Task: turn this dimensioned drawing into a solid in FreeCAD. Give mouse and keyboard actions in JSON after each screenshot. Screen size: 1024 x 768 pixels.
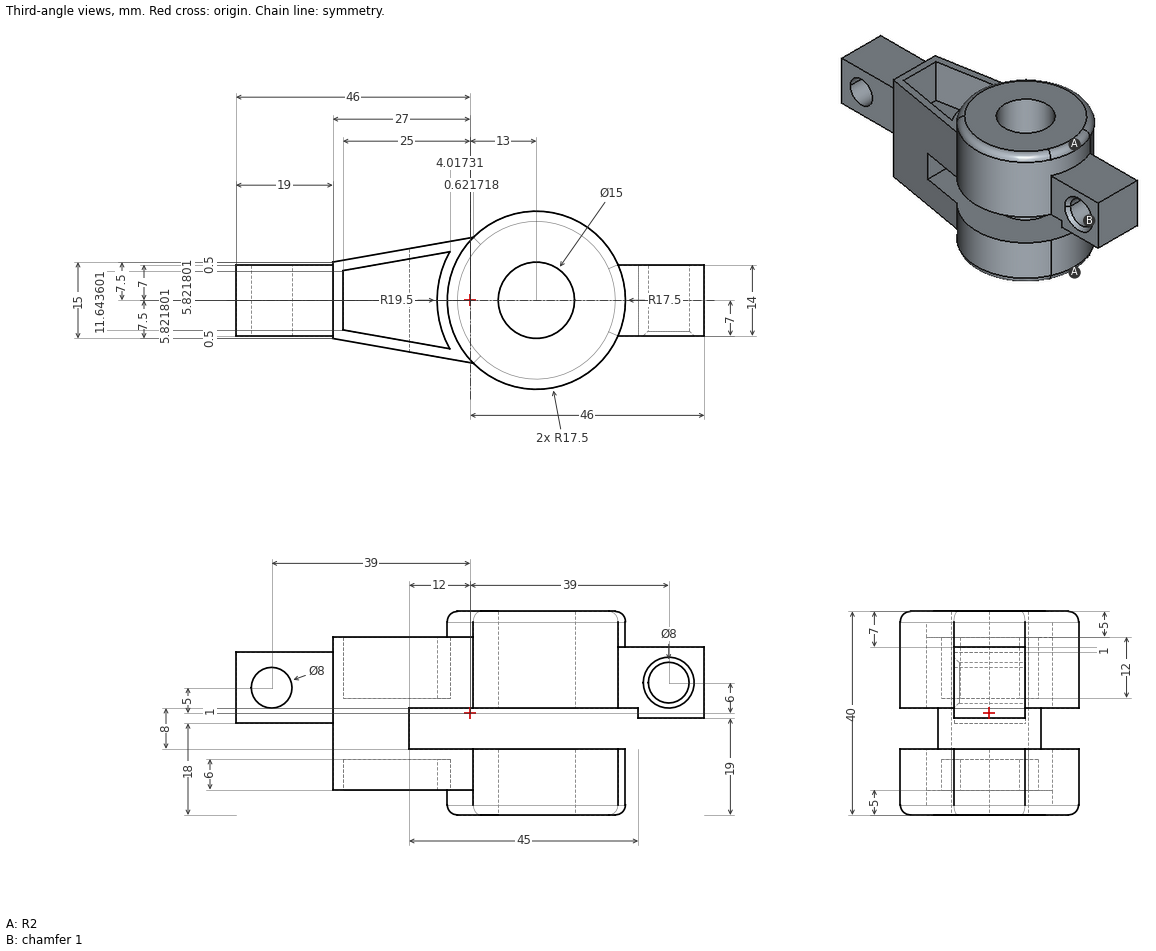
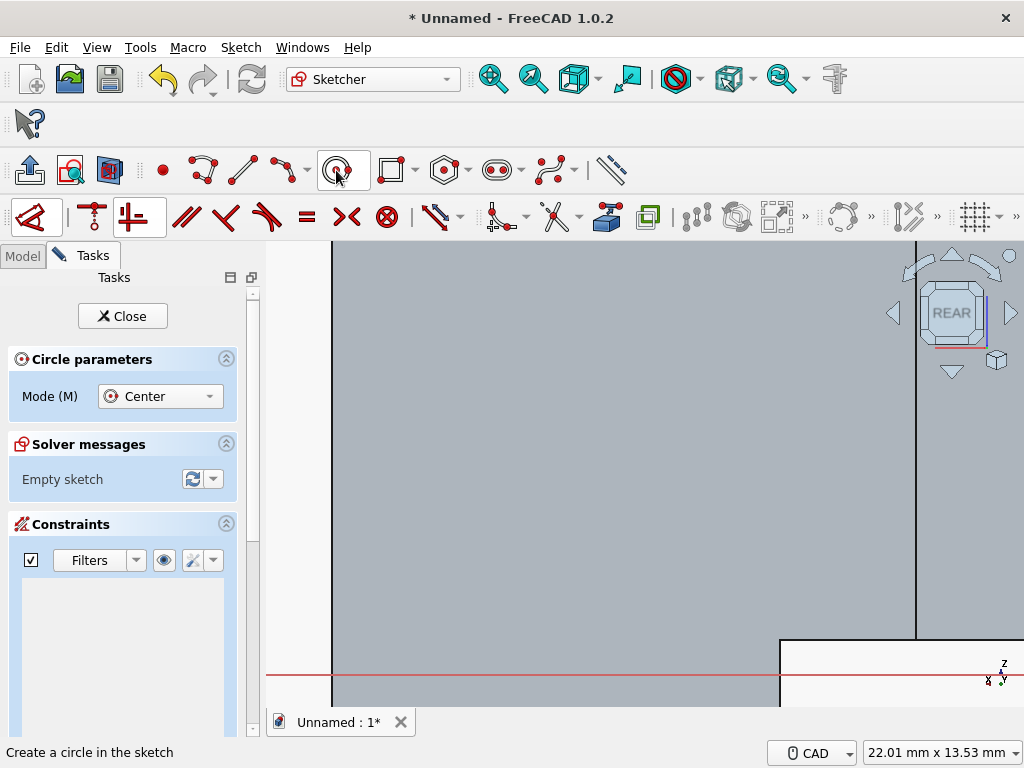
{"action": "left_click", "coordinate": [573, 468]}
{"action": "left_click", "coordinate": [670, 371]}
{"action": "key", "text": "Escape"}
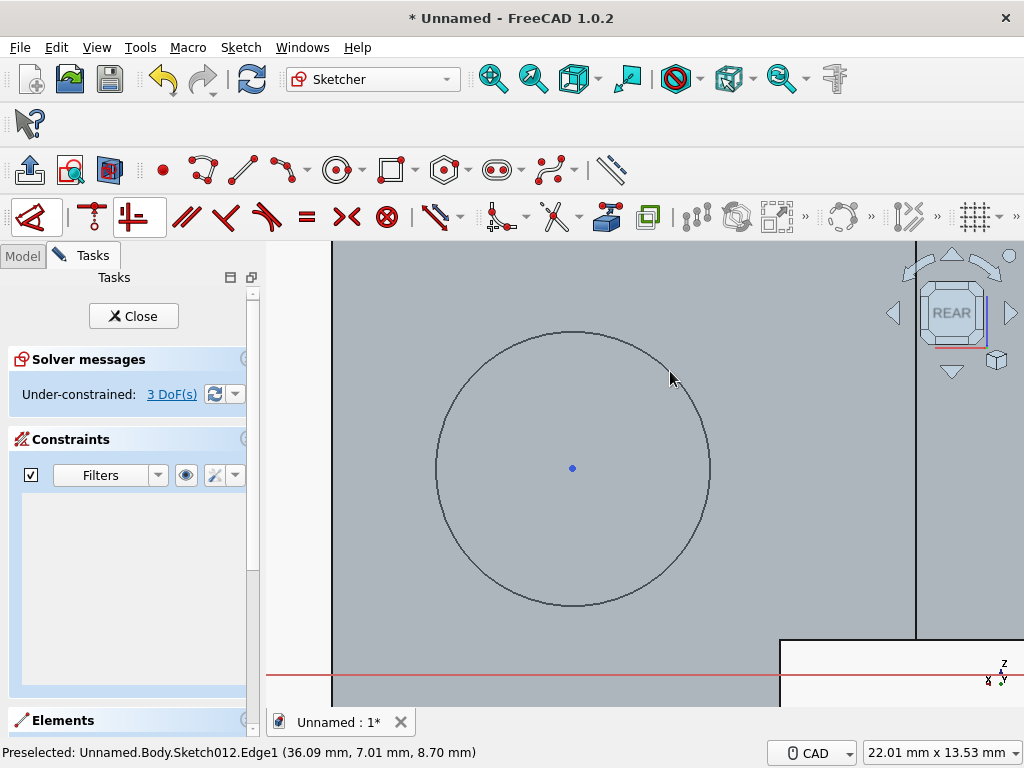
{"action": "left_click", "coordinate": [670, 372]}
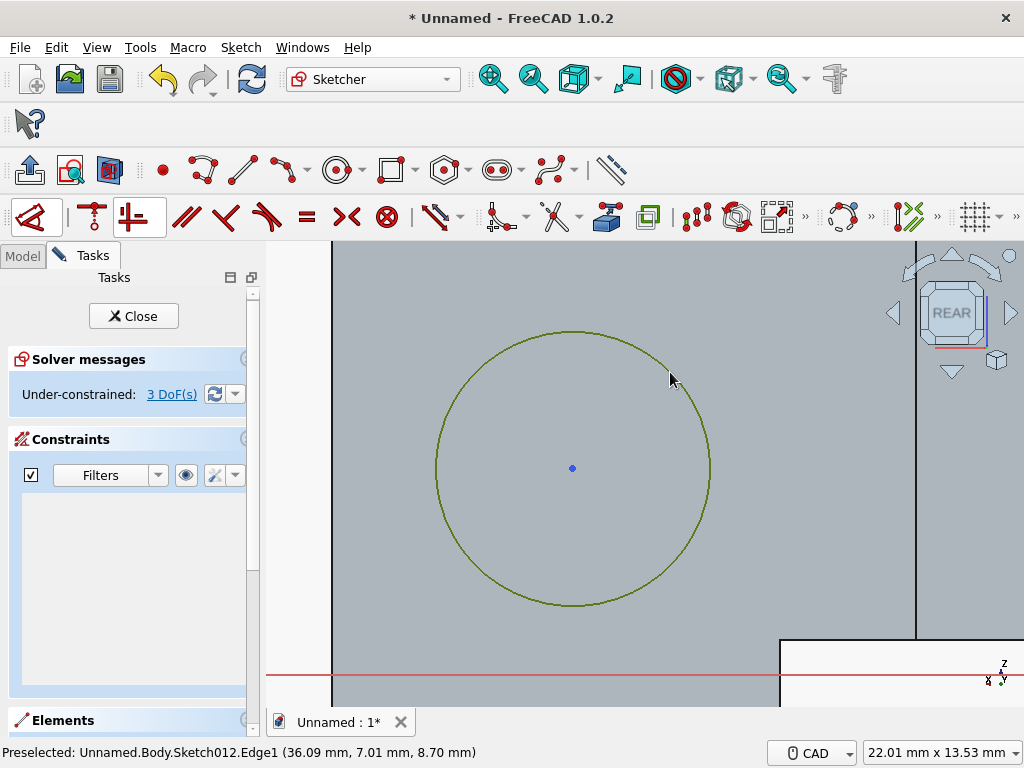
{"action": "key", "text": "k o"}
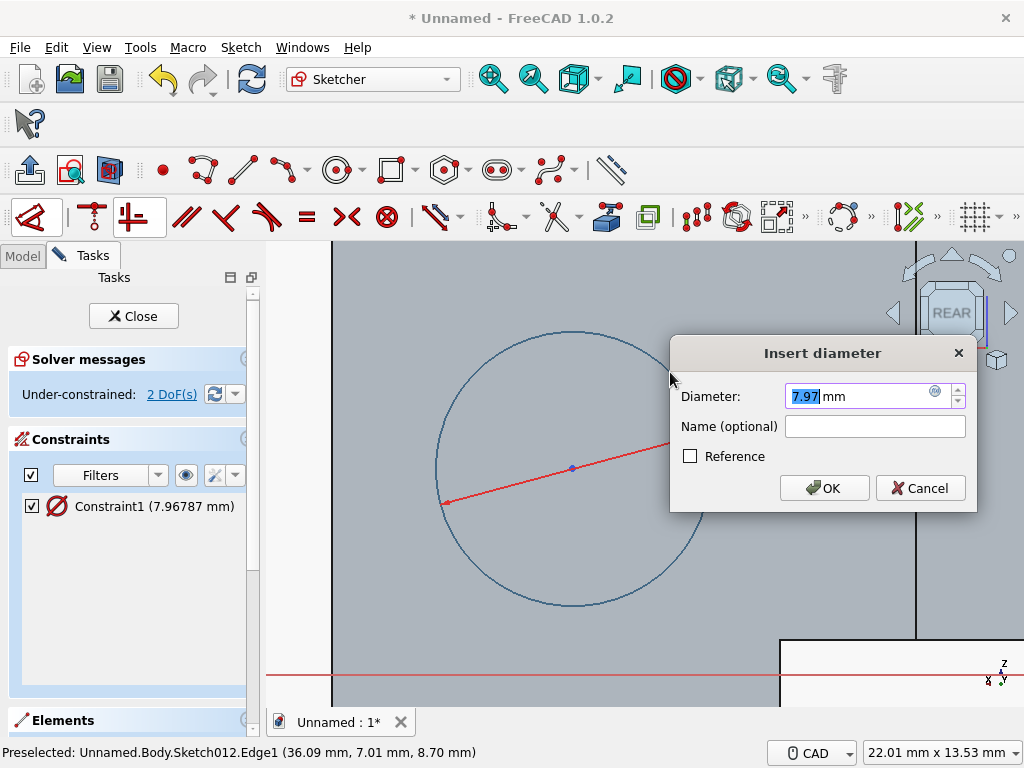
{"action": "type", "text": "8"}
{"action": "key", "text": "Return"}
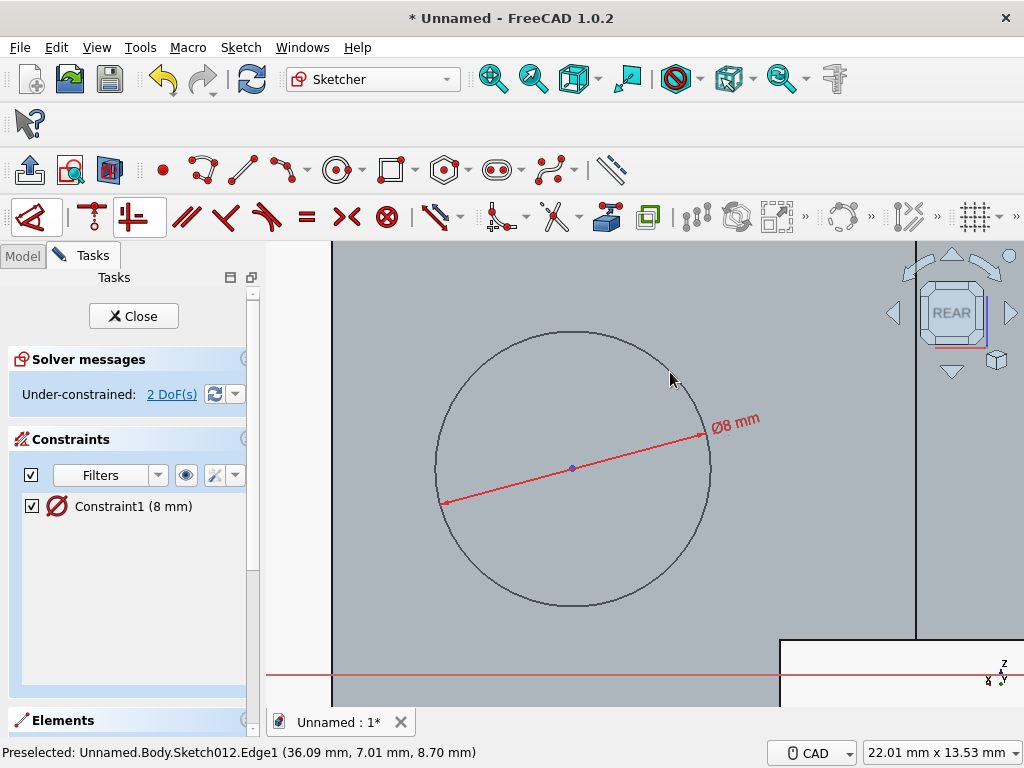
{"action": "left_click", "coordinate": [573, 469]}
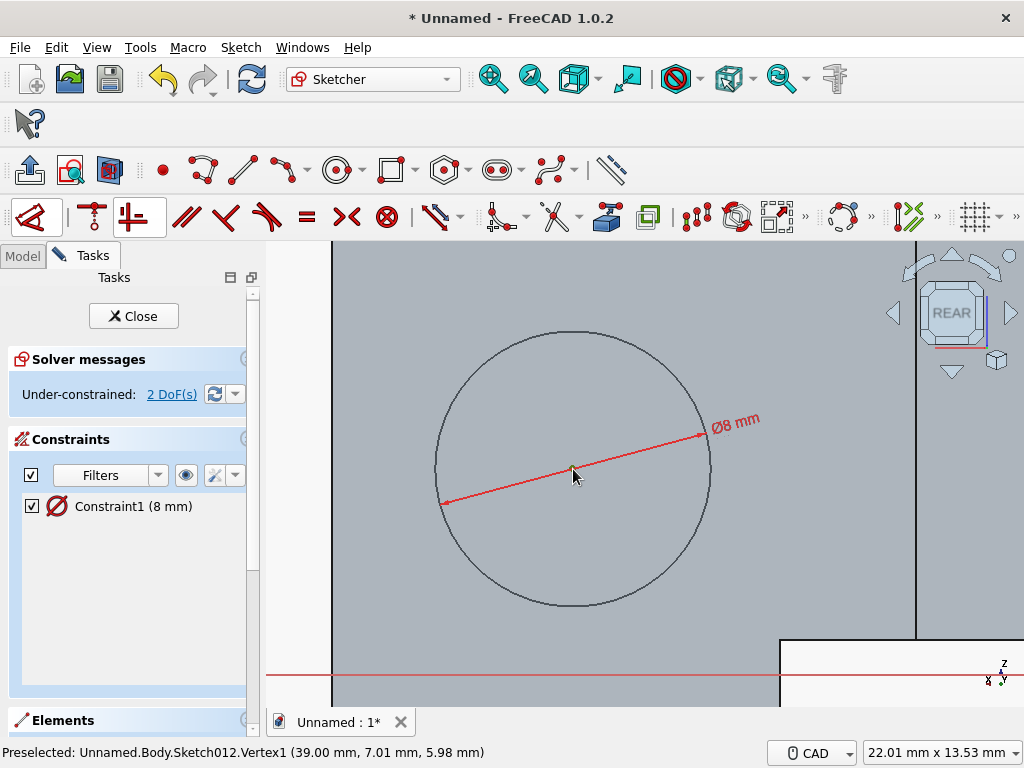
{"action": "key", "text": "i"}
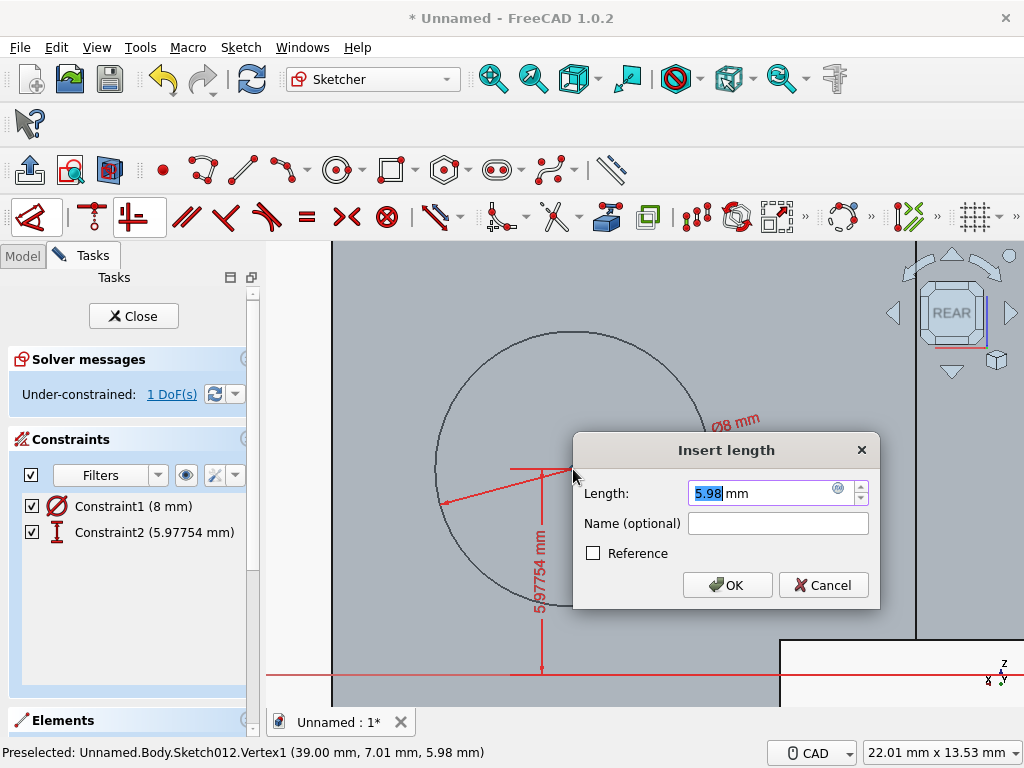
{"action": "type", "text": "6"}
{"action": "key", "text": "Return"}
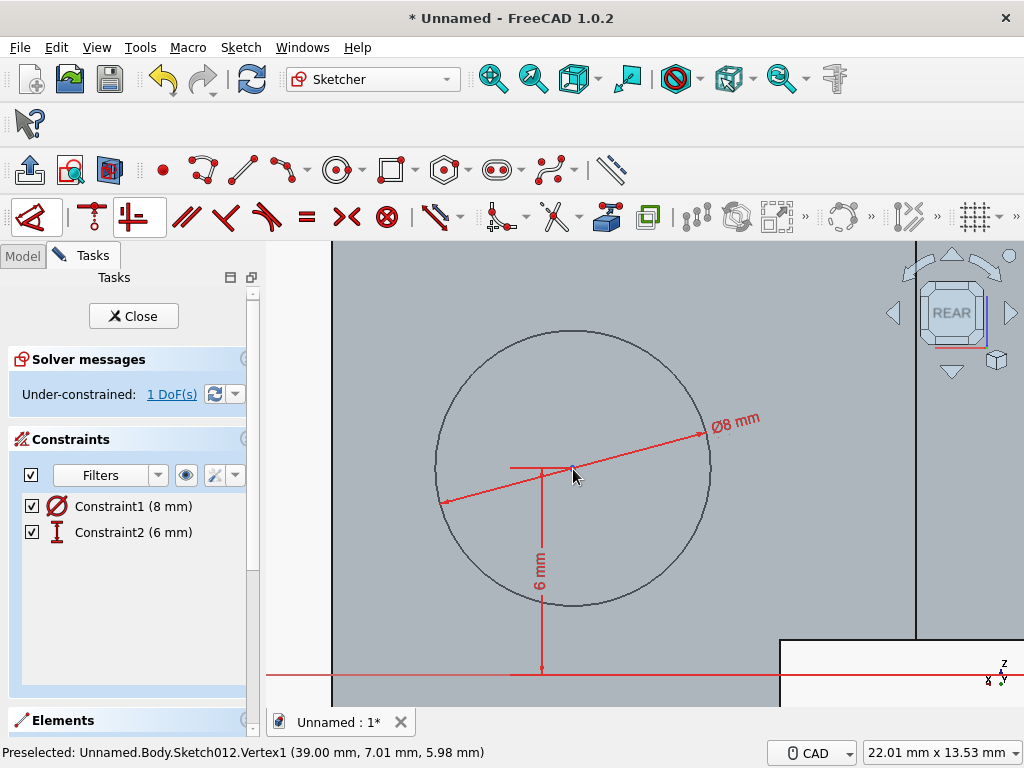
{"action": "left_click", "coordinate": [573, 468]}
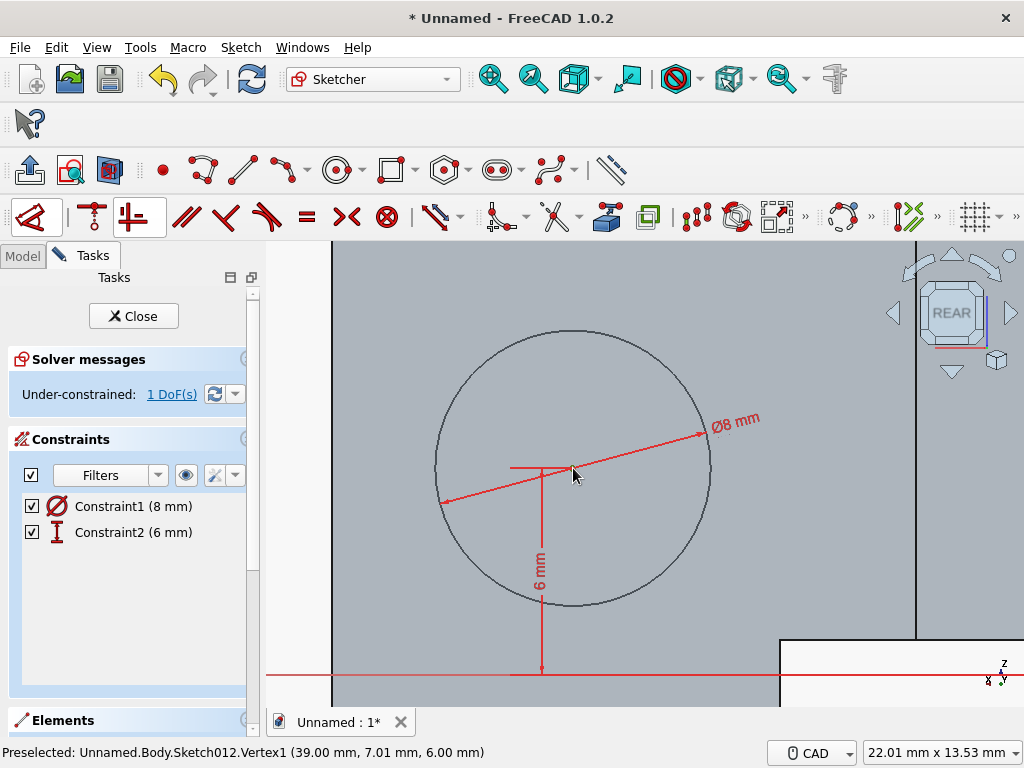
{"action": "key", "text": "l"}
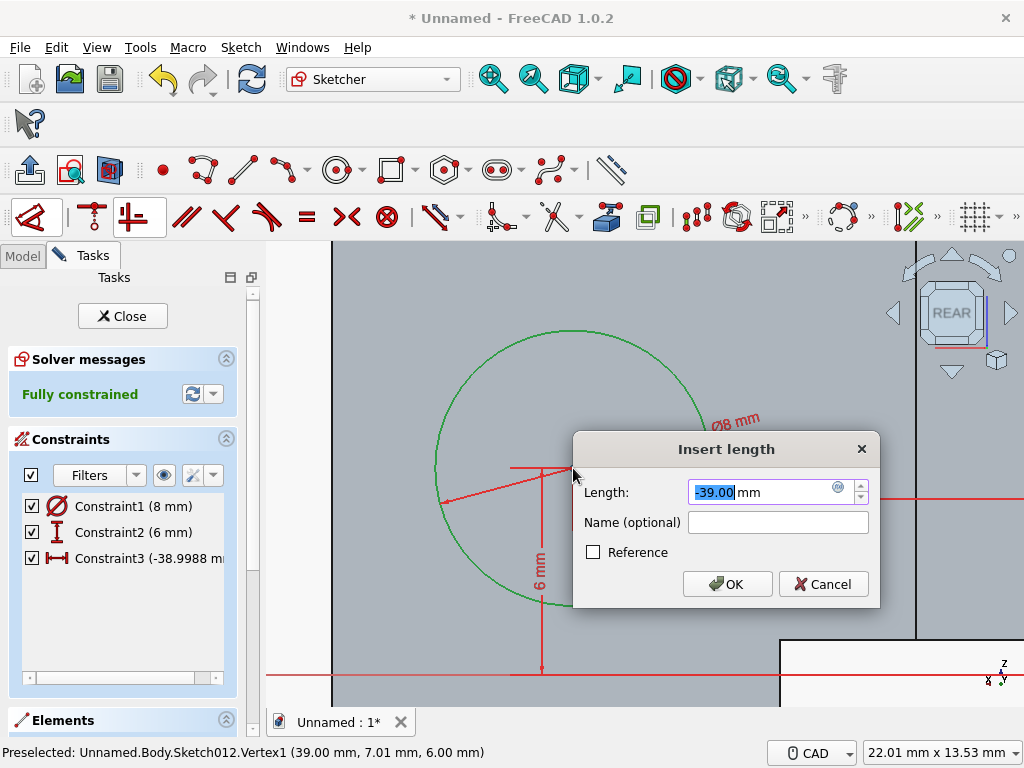
{"action": "type", "text": "-39"}
{"action": "key", "text": "Return"}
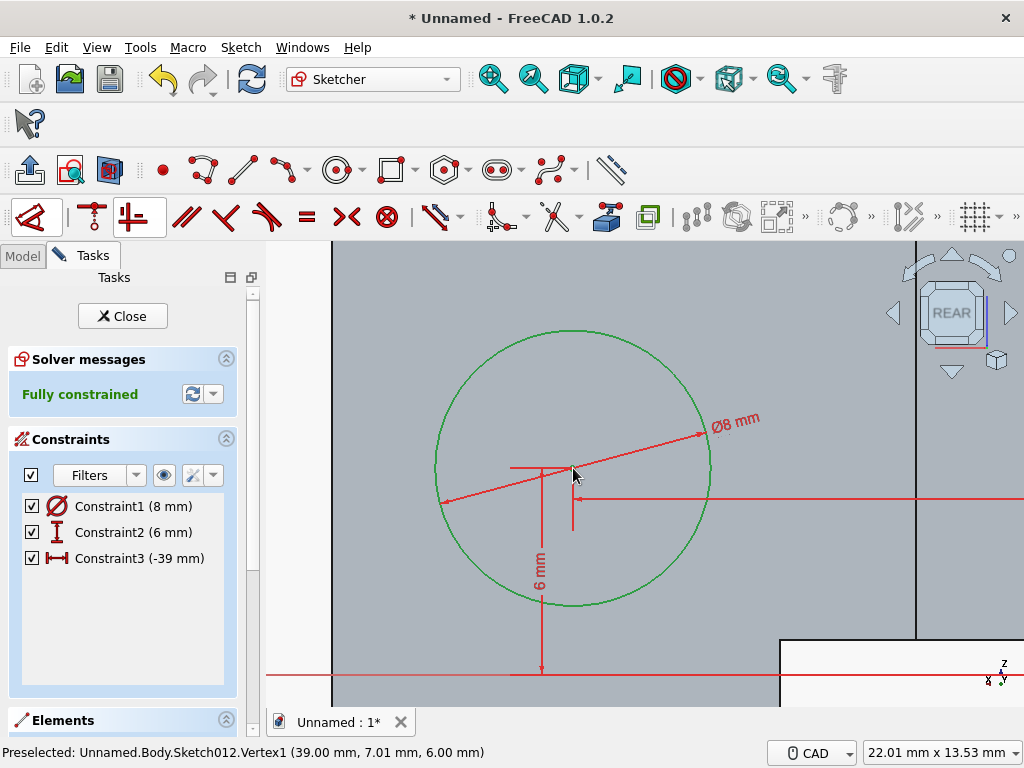
{"action": "left_click", "coordinate": [123, 316]}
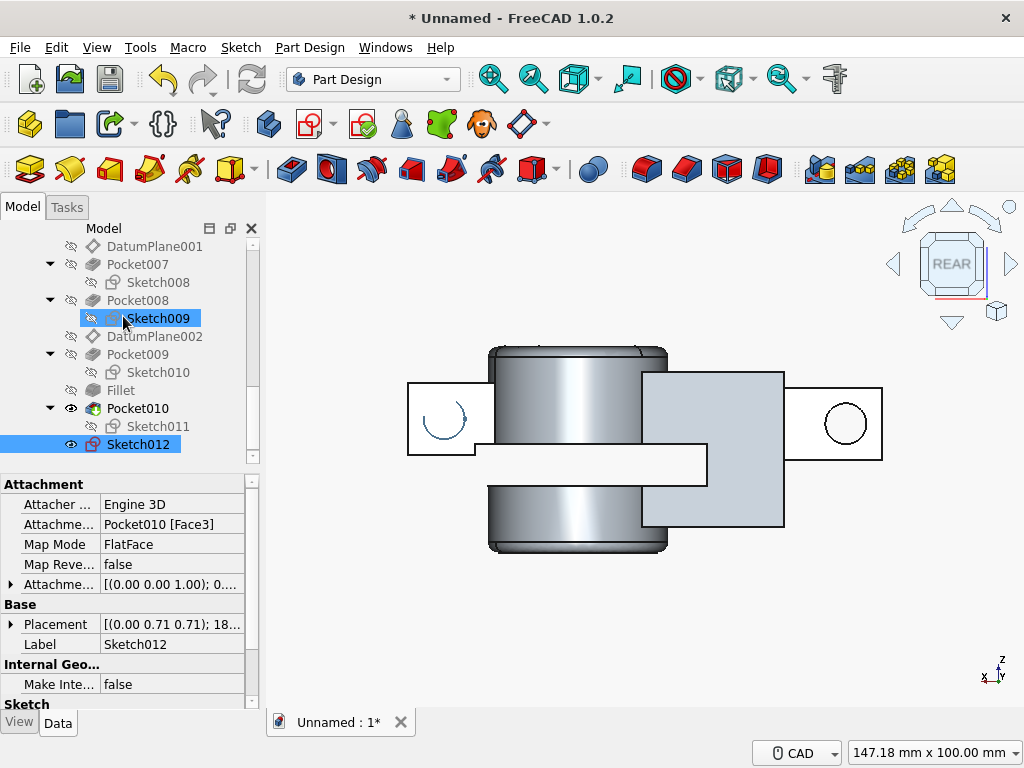
{"action": "left_click", "coordinate": [292, 170]}